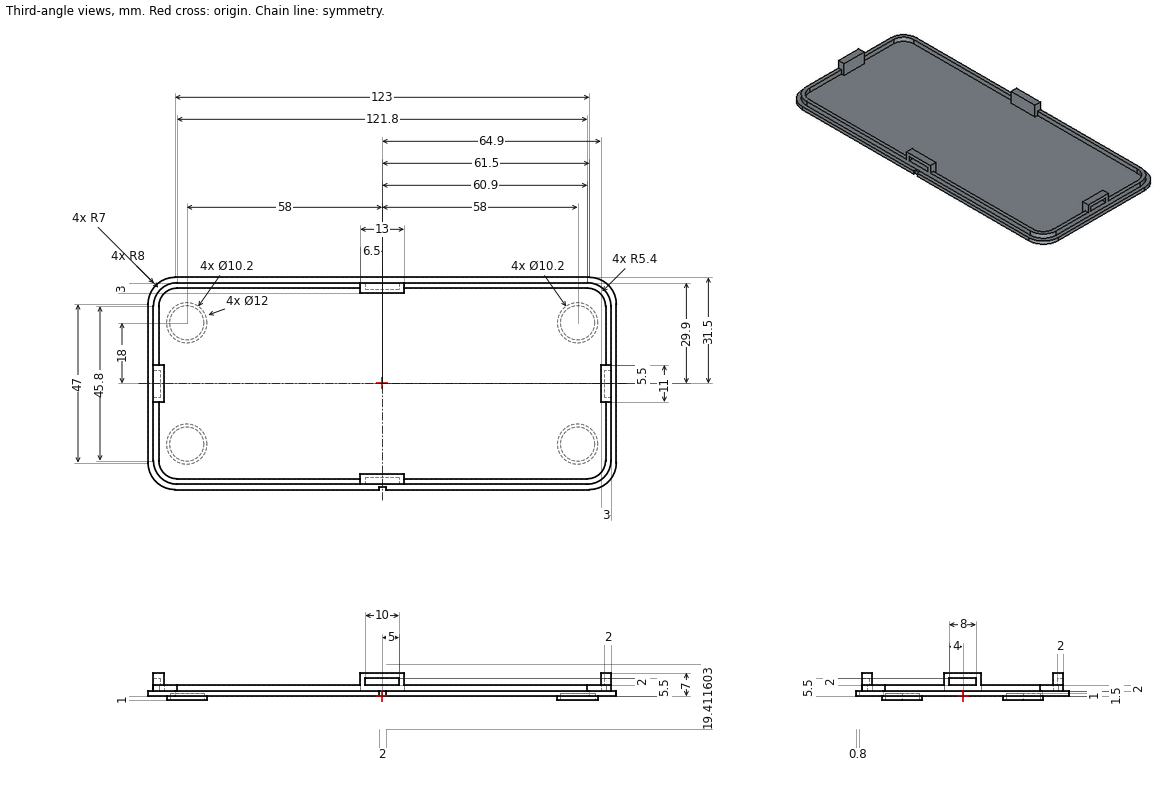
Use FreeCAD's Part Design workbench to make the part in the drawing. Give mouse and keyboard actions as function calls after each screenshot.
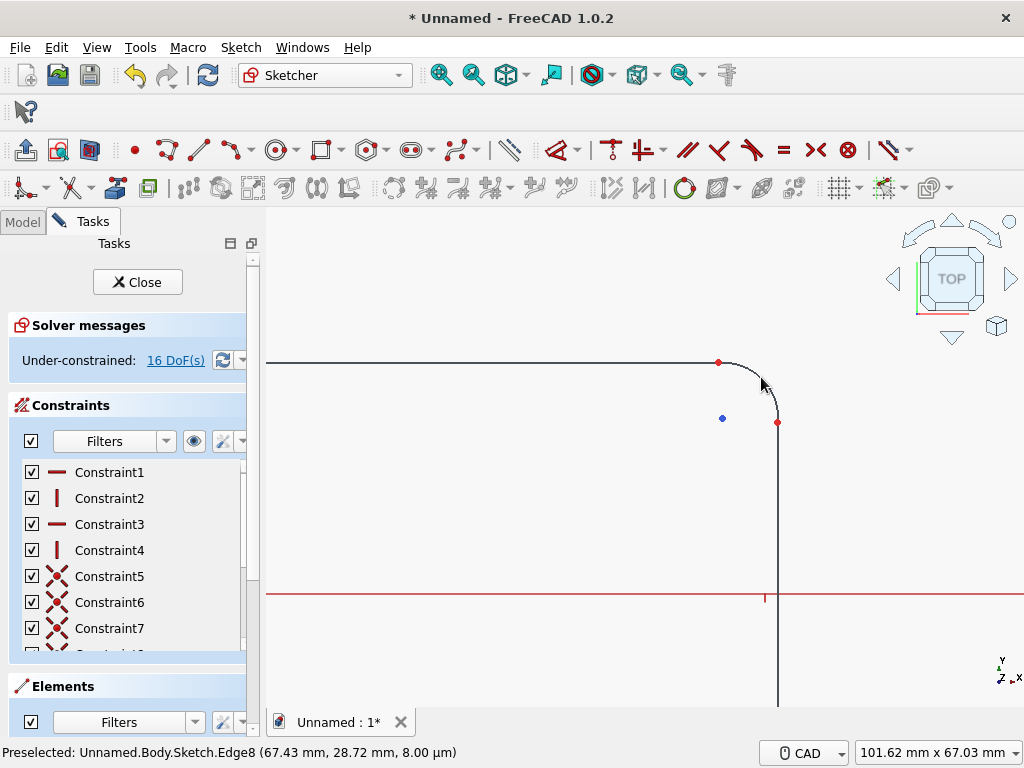
click(443, 363)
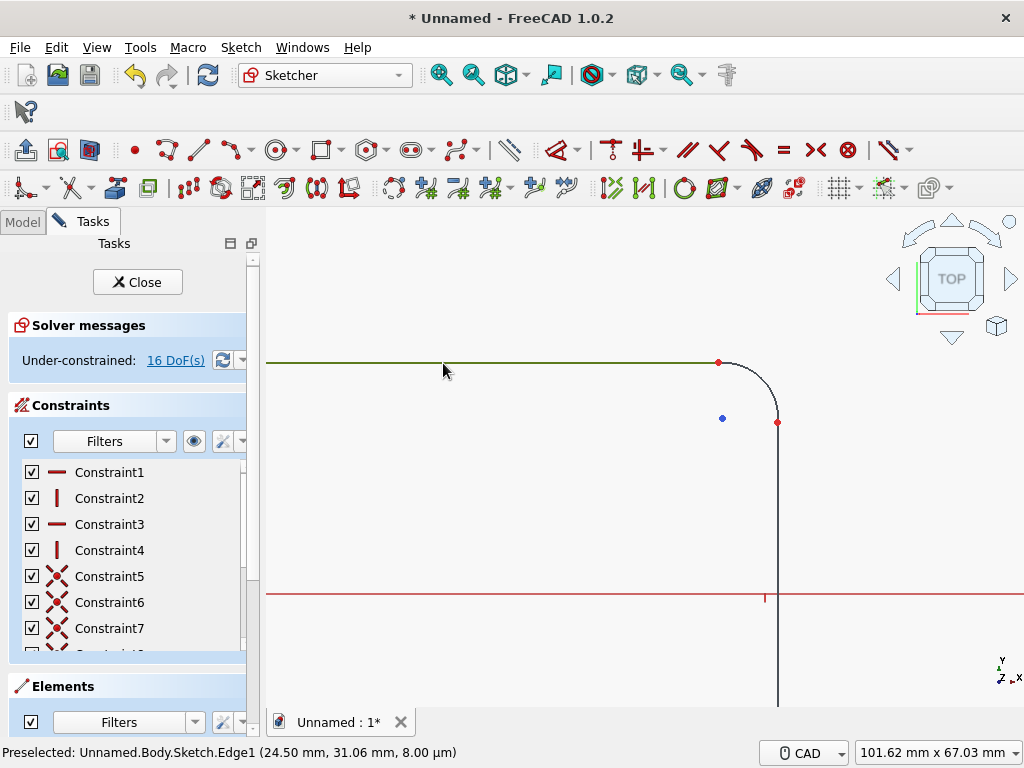
scroll(761, 377, down, 5)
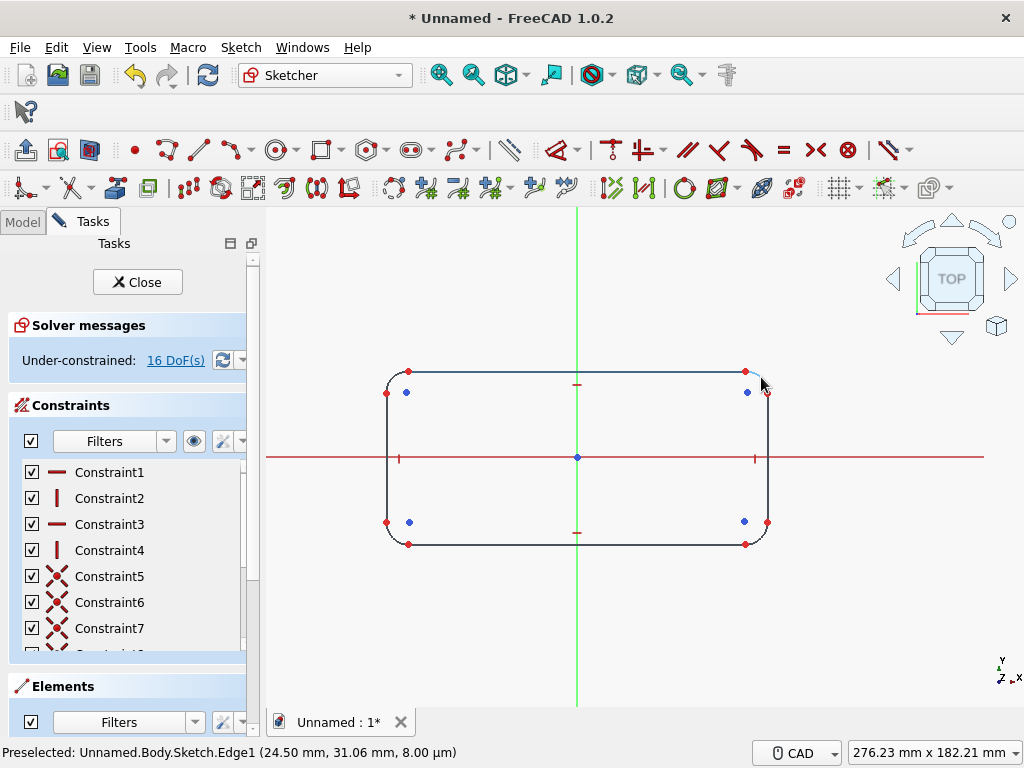
scroll(398, 374, up, 2)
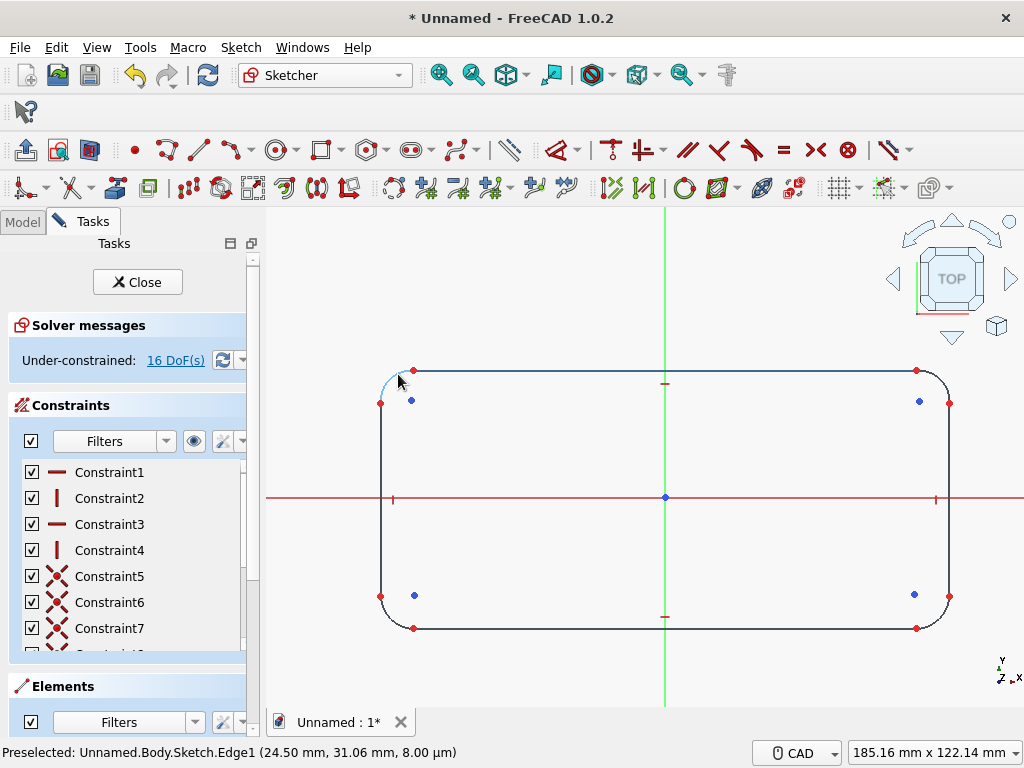
click(398, 374)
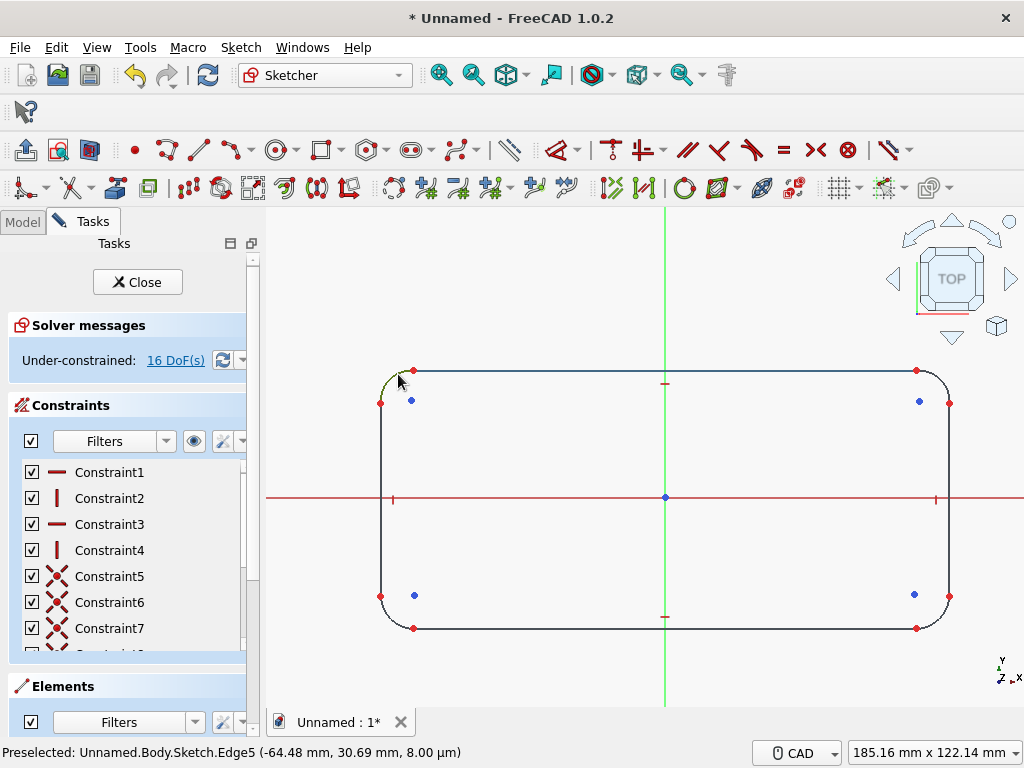
key(t)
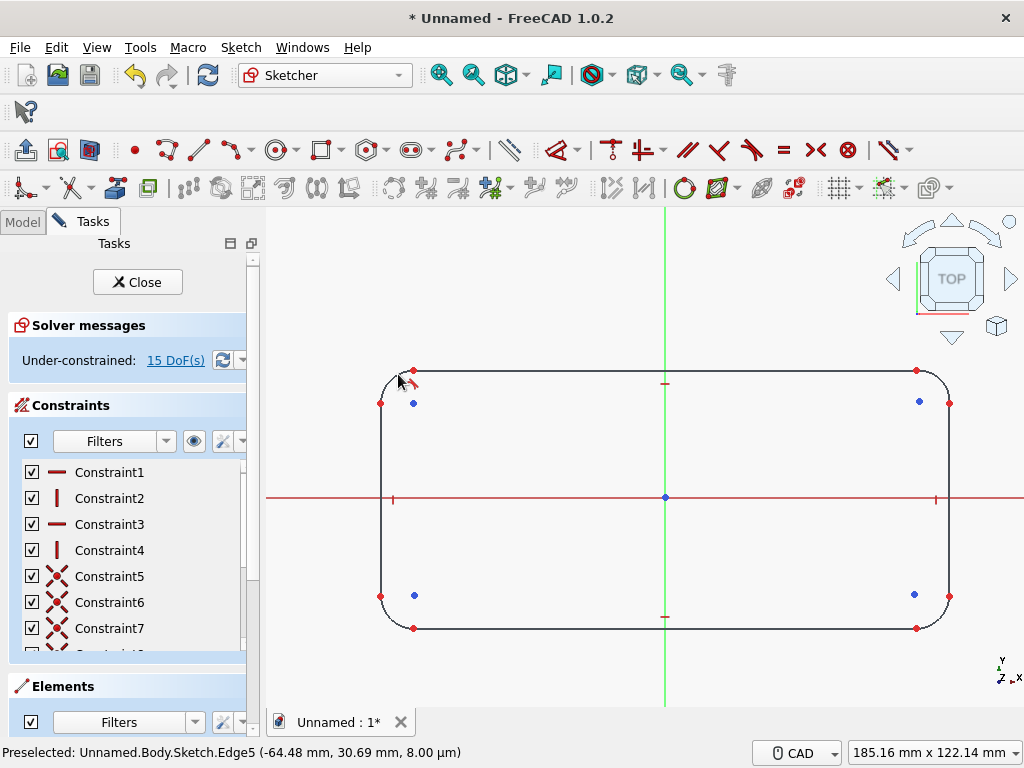
click(766, 371)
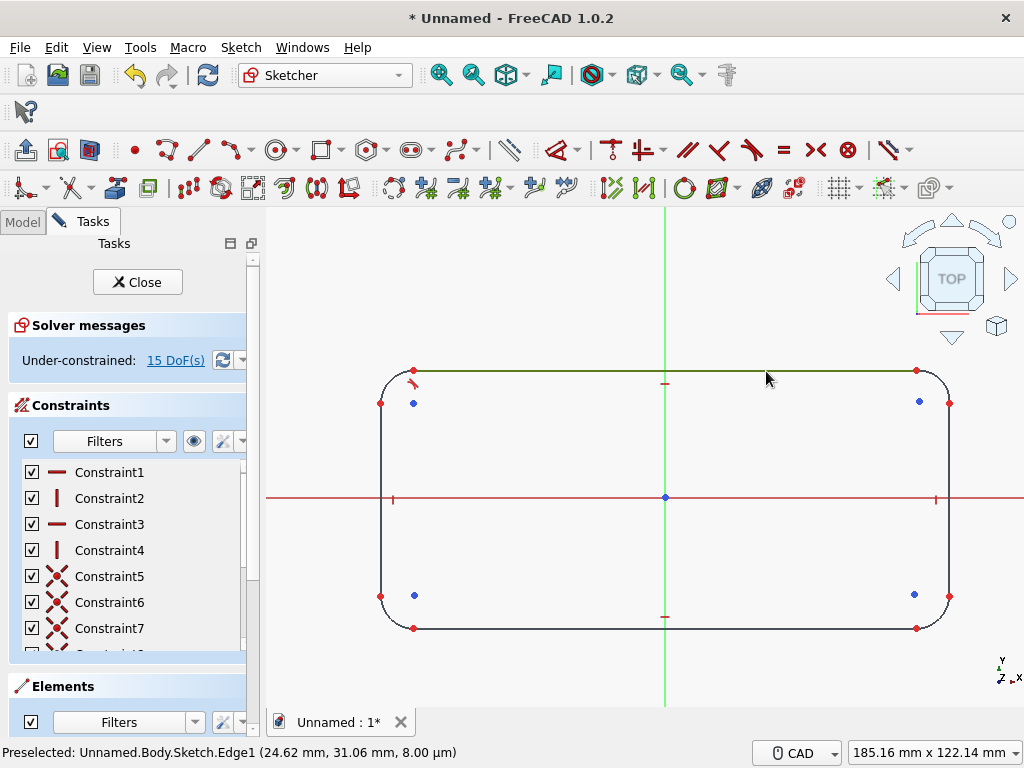
scroll(396, 374, down, 2)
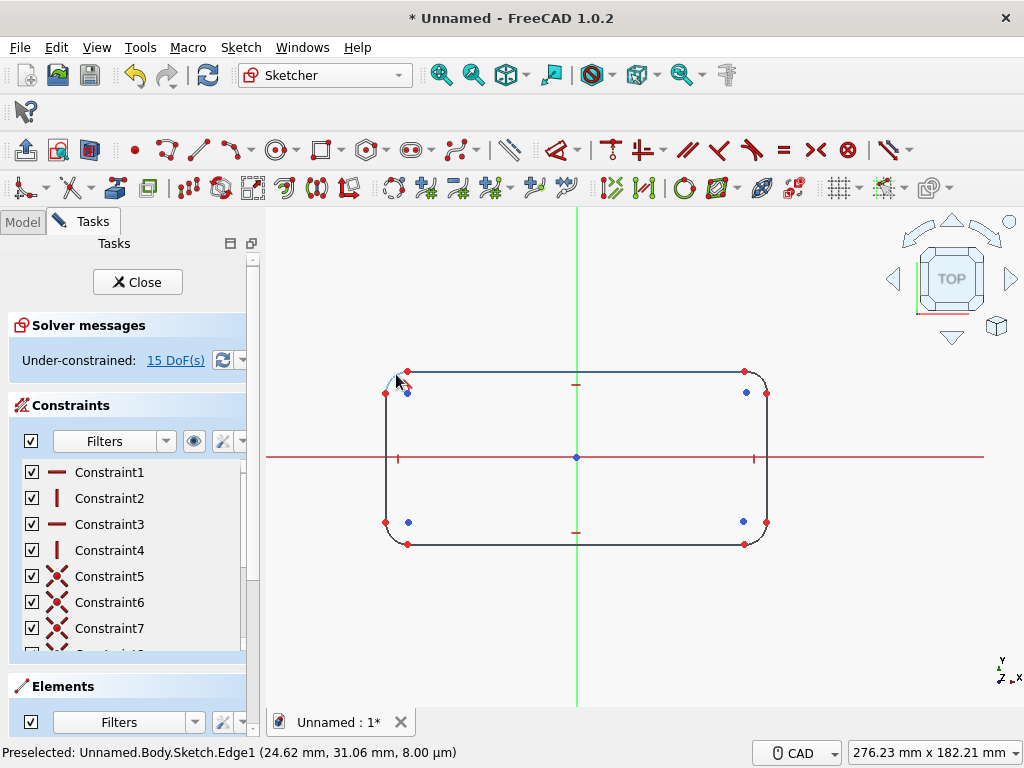
scroll(765, 384, up, 2)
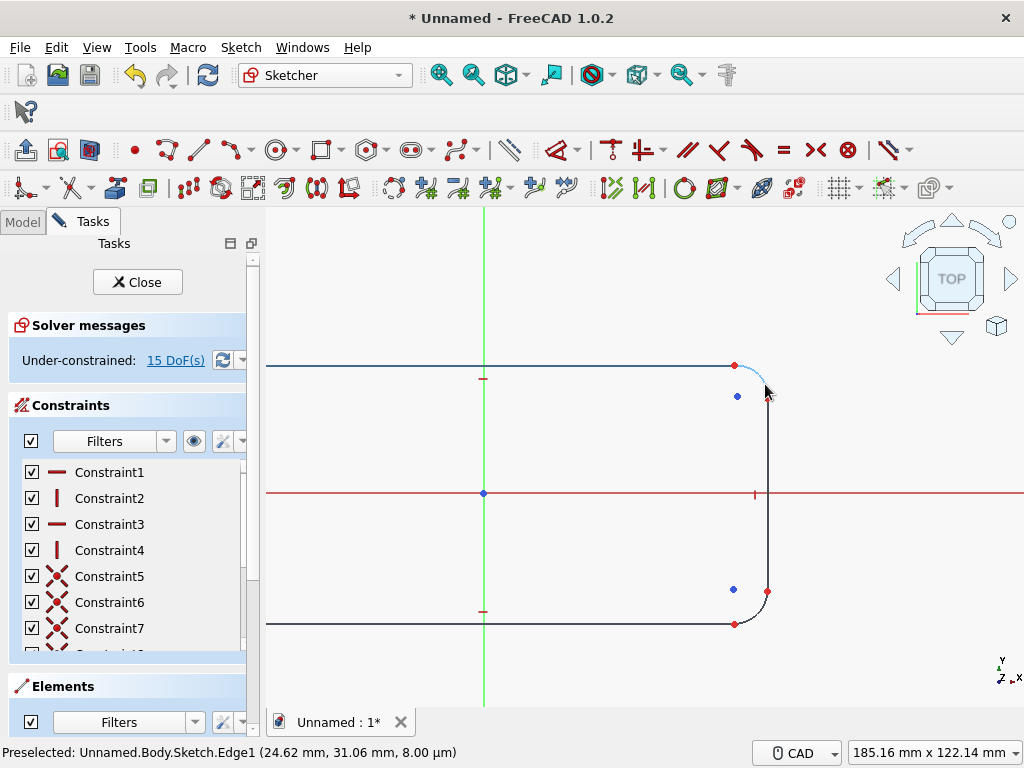
click(765, 383)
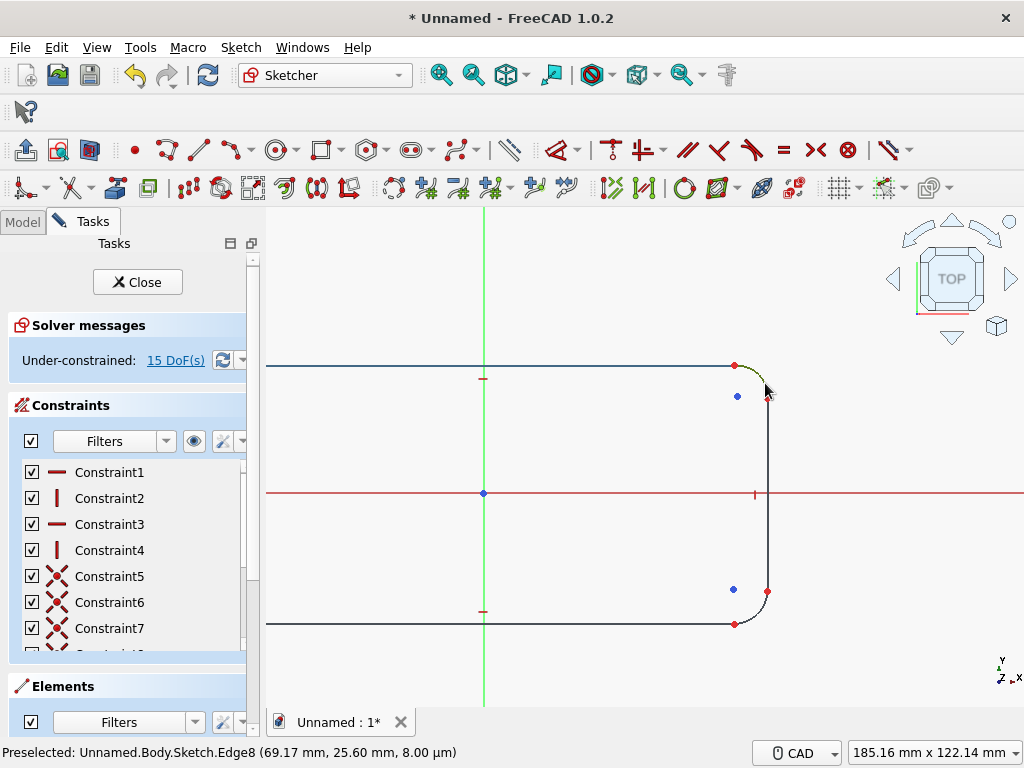
key(t)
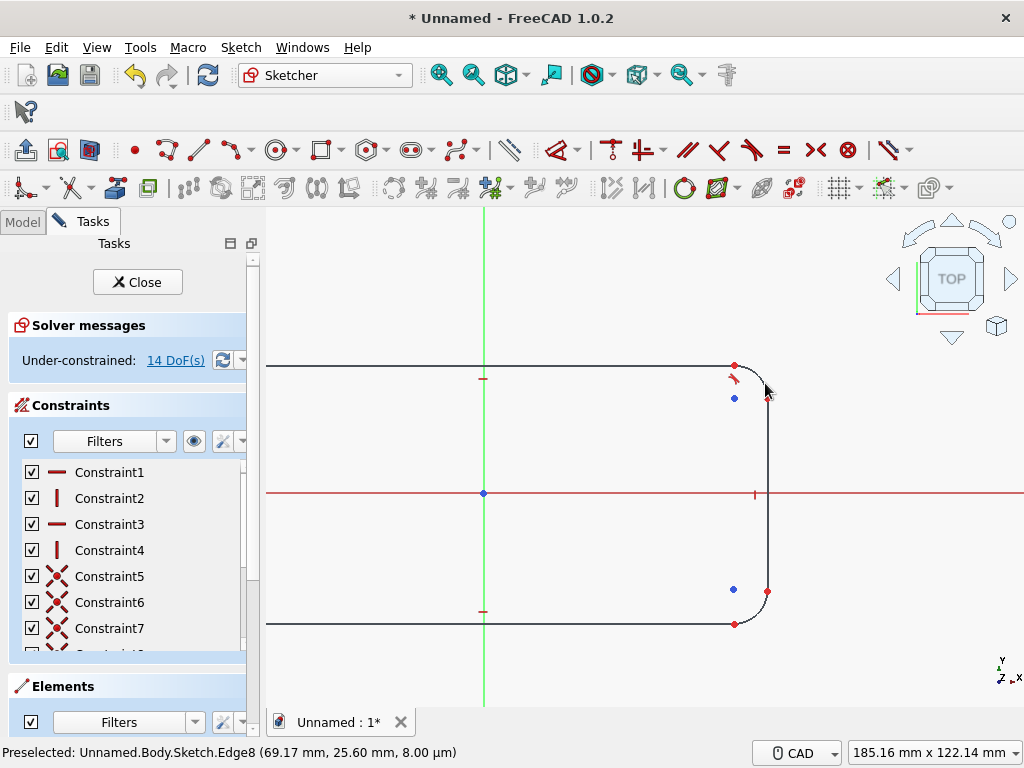
scroll(766, 384, down, 2)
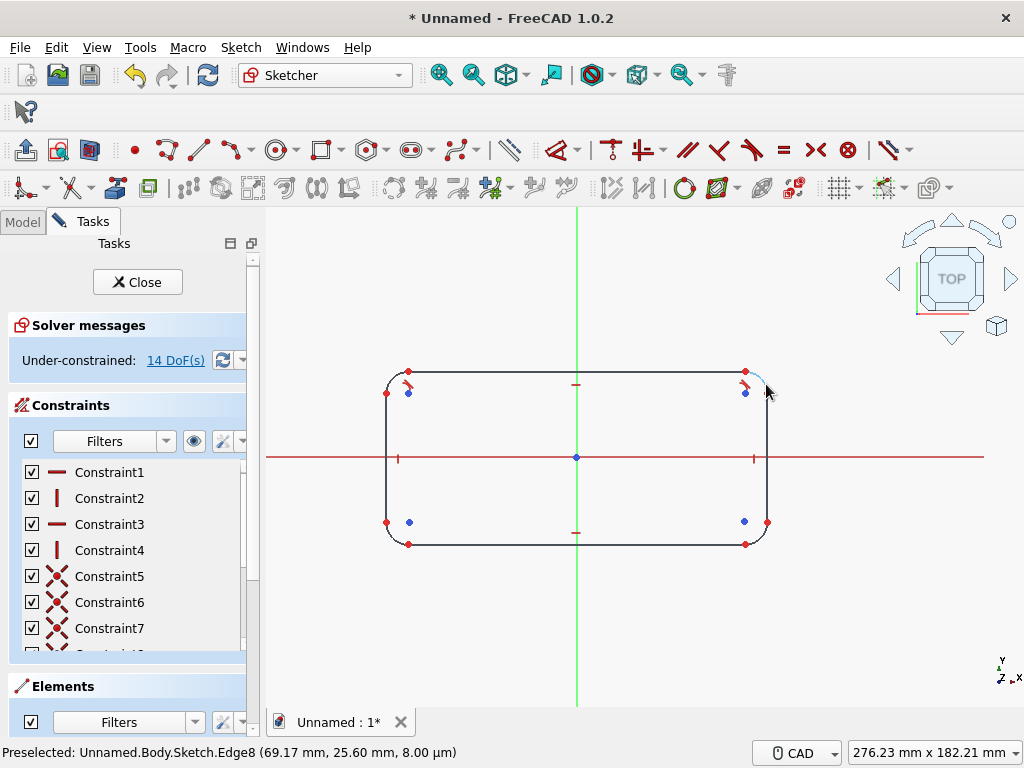
click(386, 433)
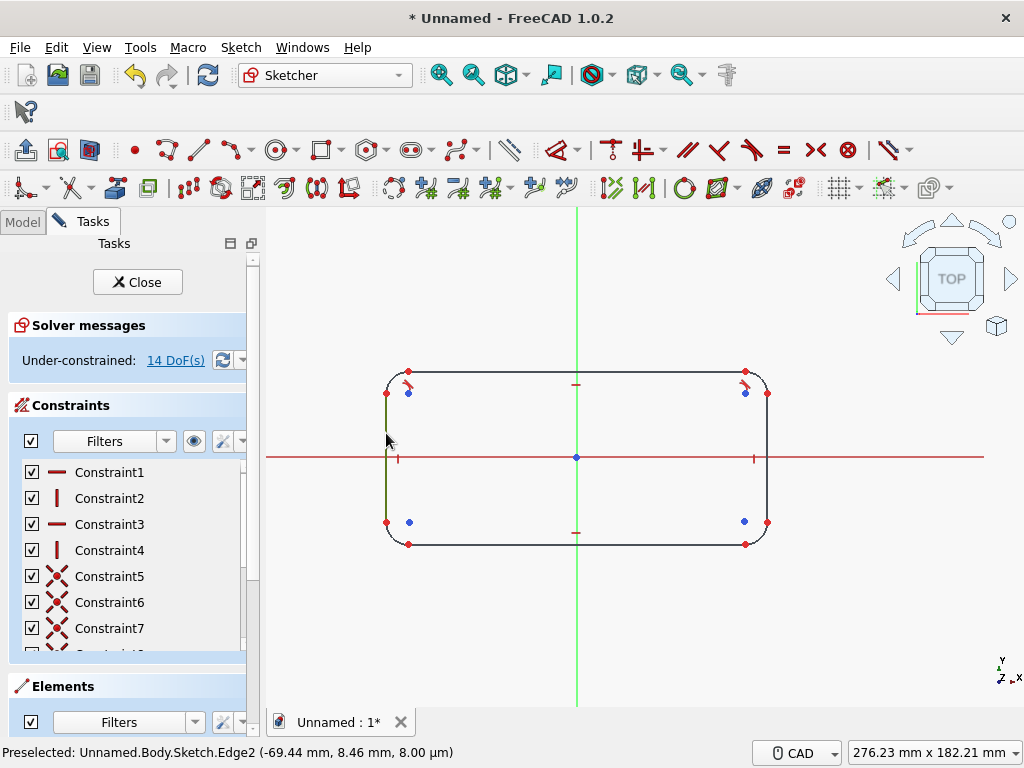
scroll(398, 374, up, 2)